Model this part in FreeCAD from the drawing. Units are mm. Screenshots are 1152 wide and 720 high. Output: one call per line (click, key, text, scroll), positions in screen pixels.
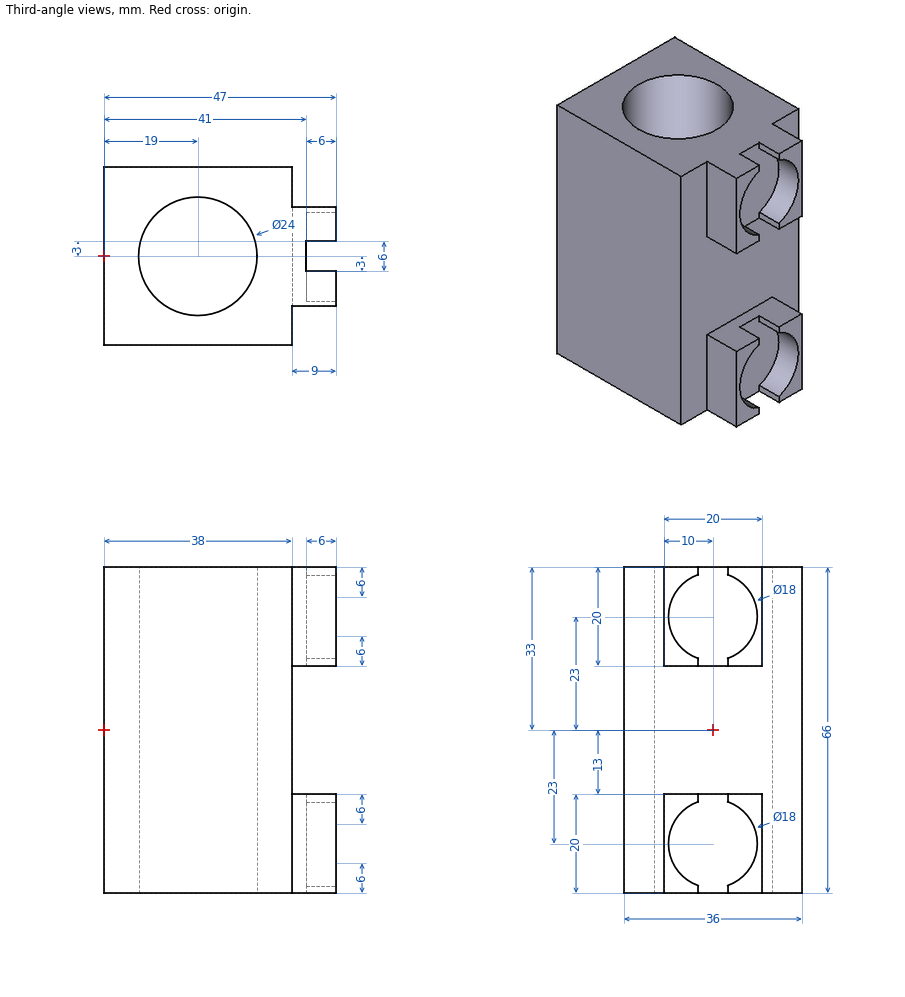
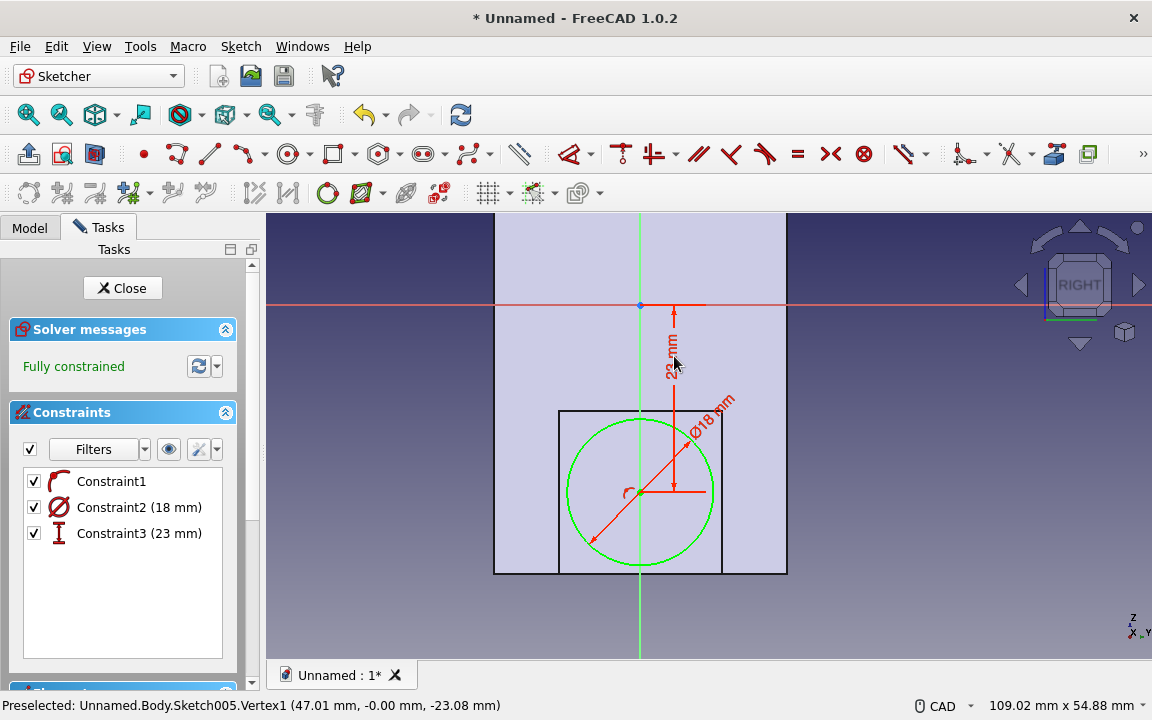
click(123, 288)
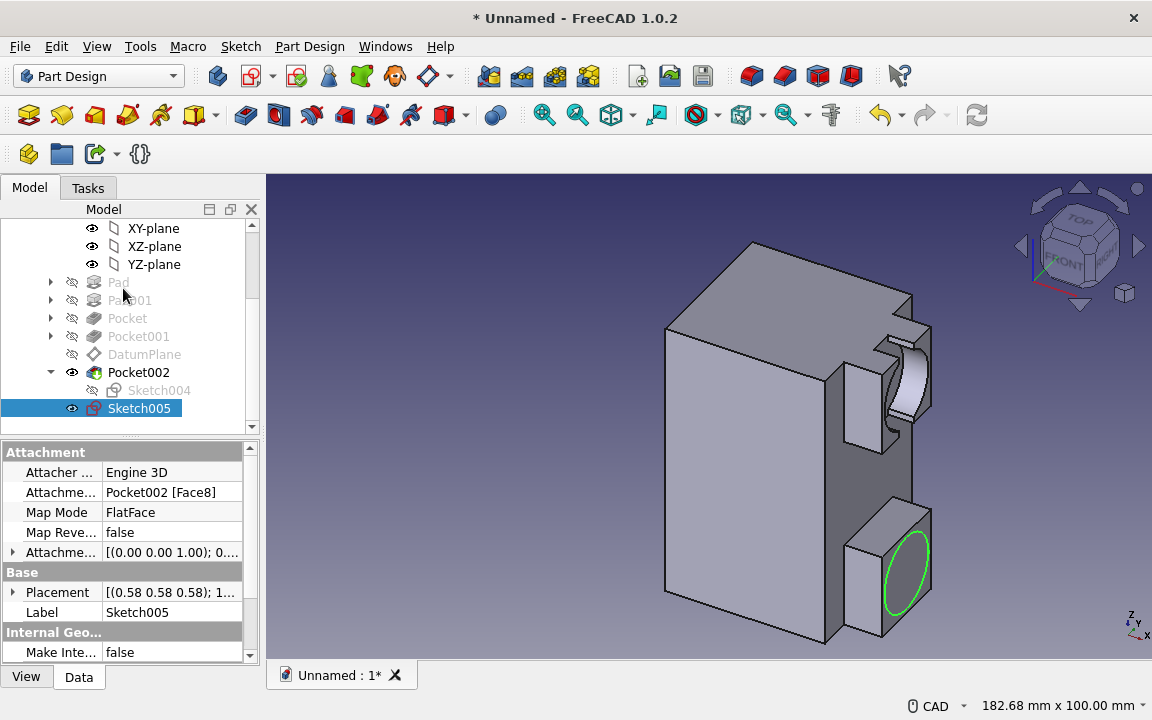
click(246, 116)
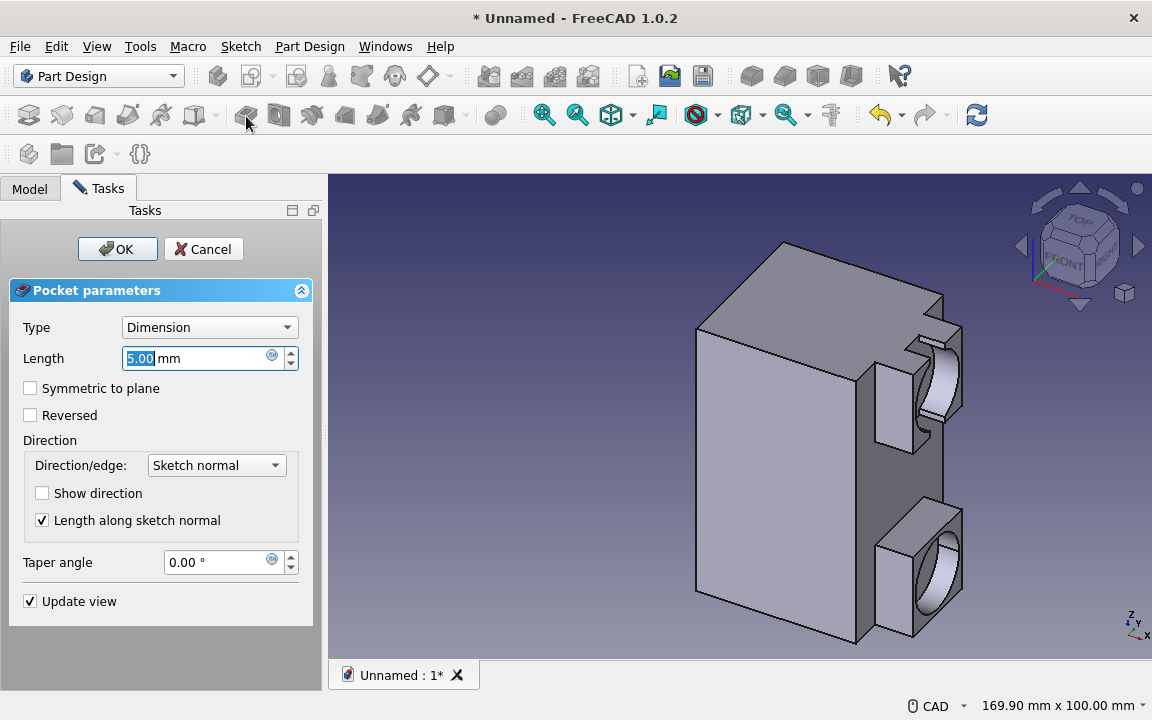
text(6)
key(Tab)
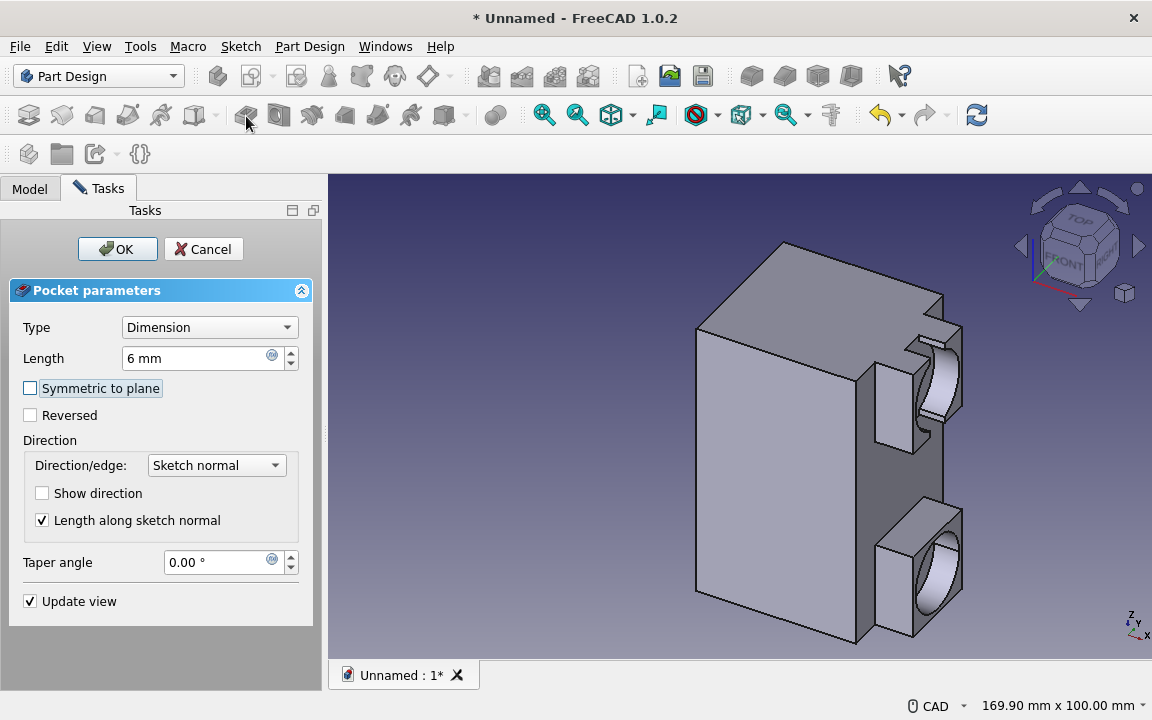
click(118, 249)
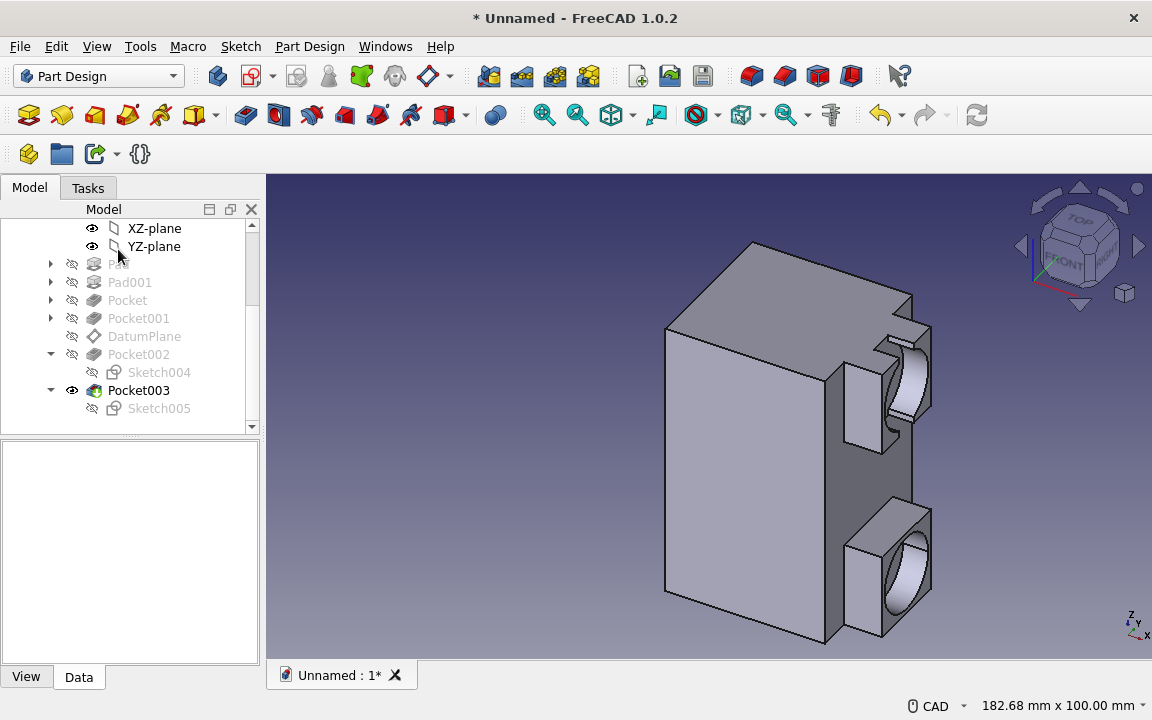
key(5)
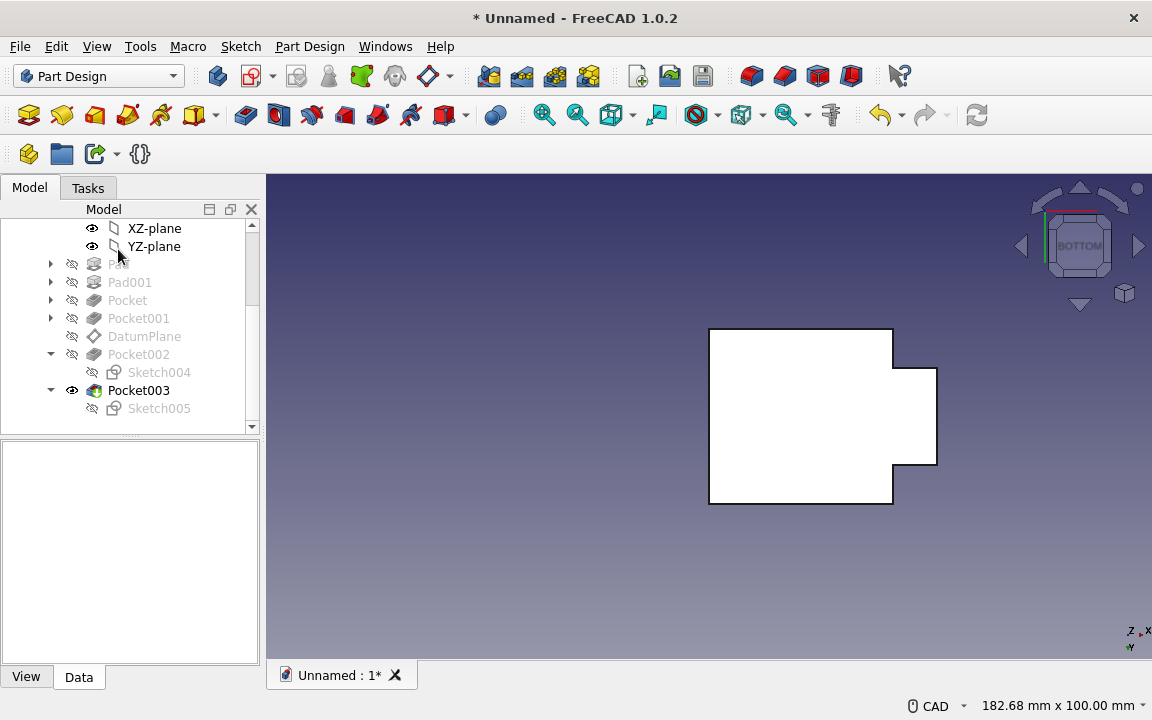
click(545, 116)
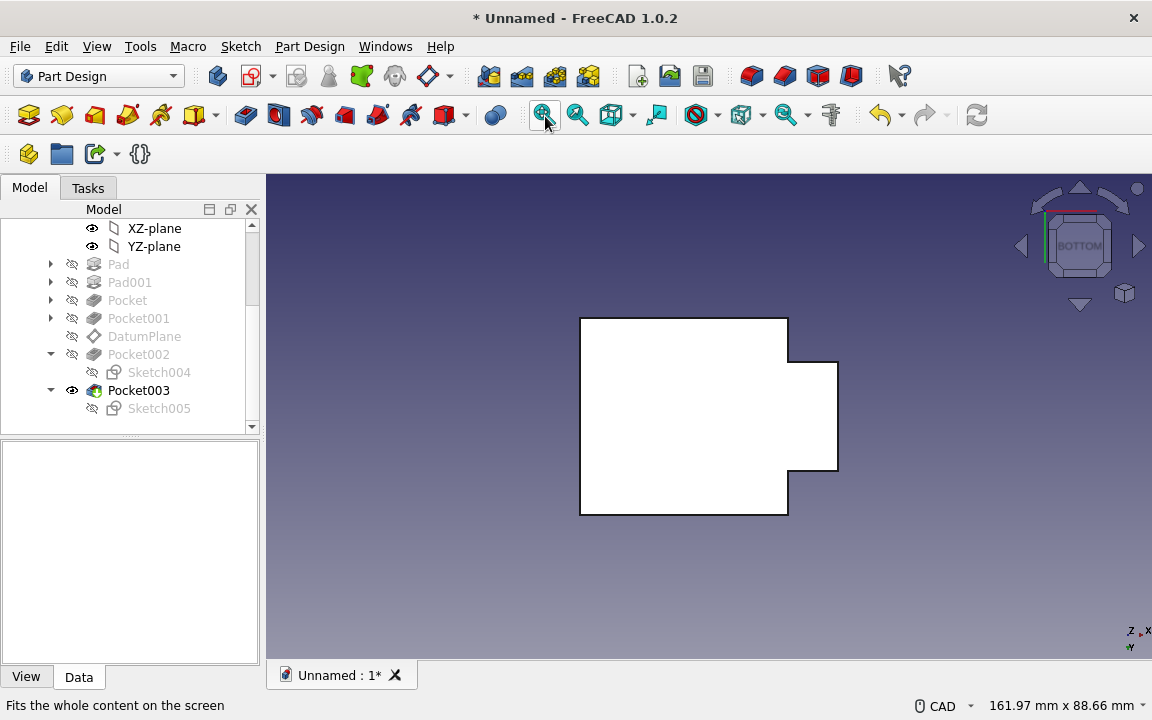
click(709, 415)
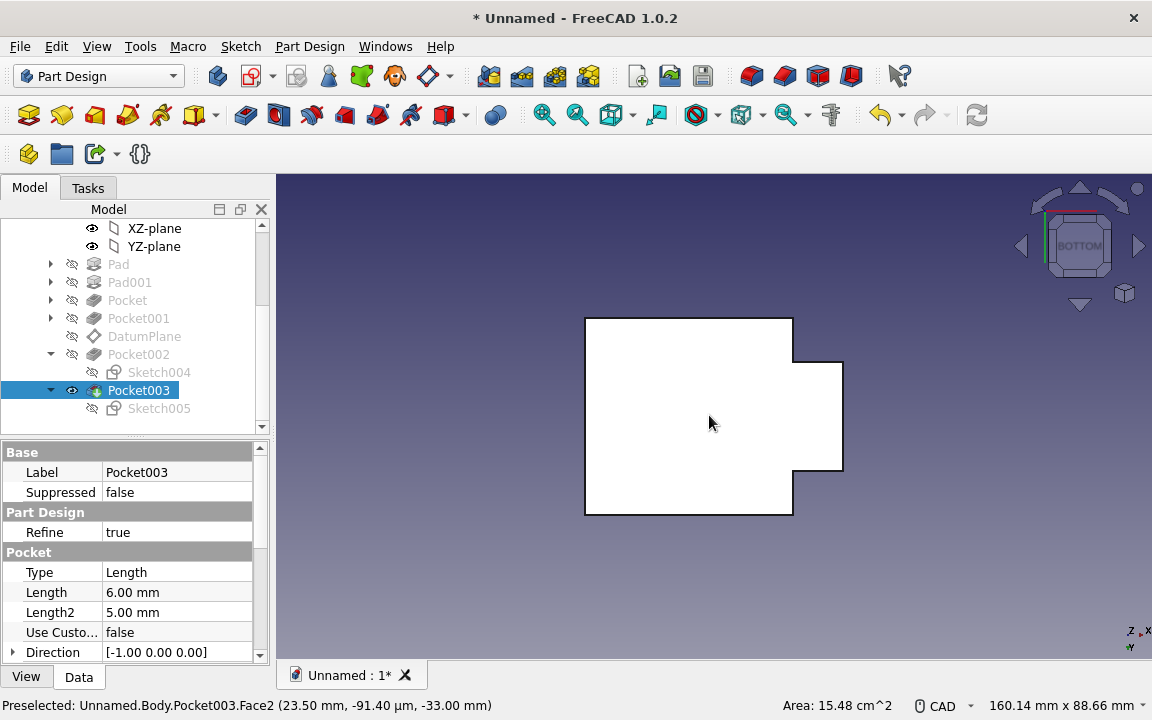
click(250, 76)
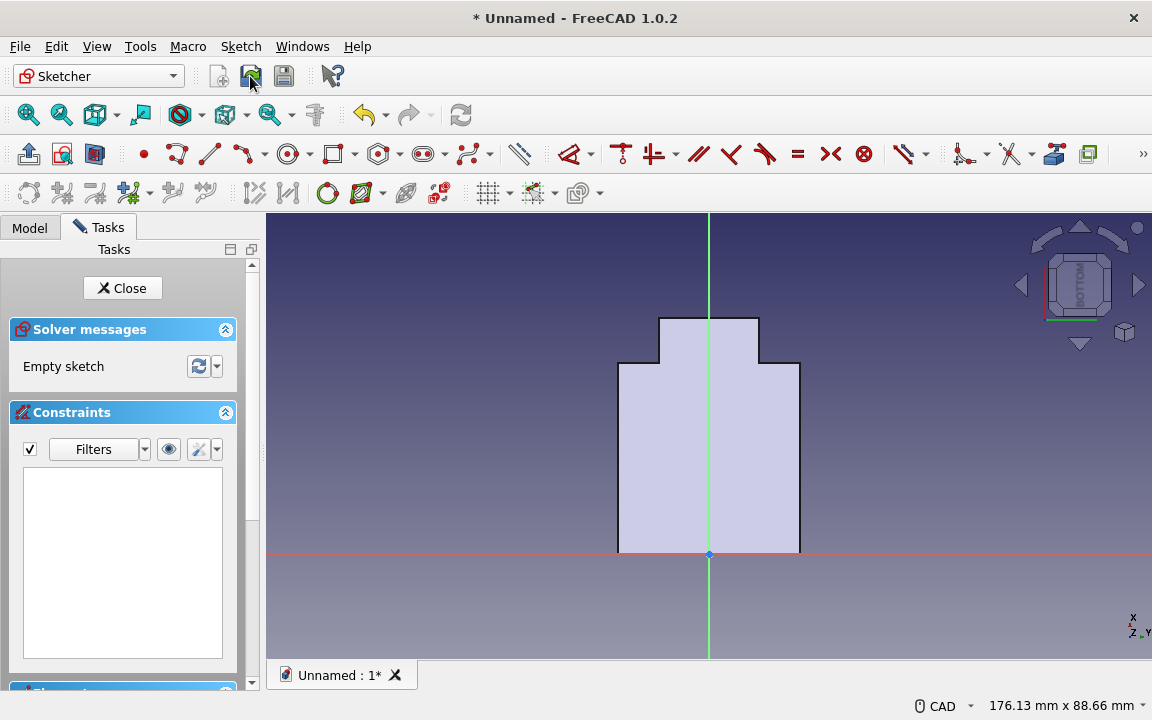
scroll(718, 320, up, 11)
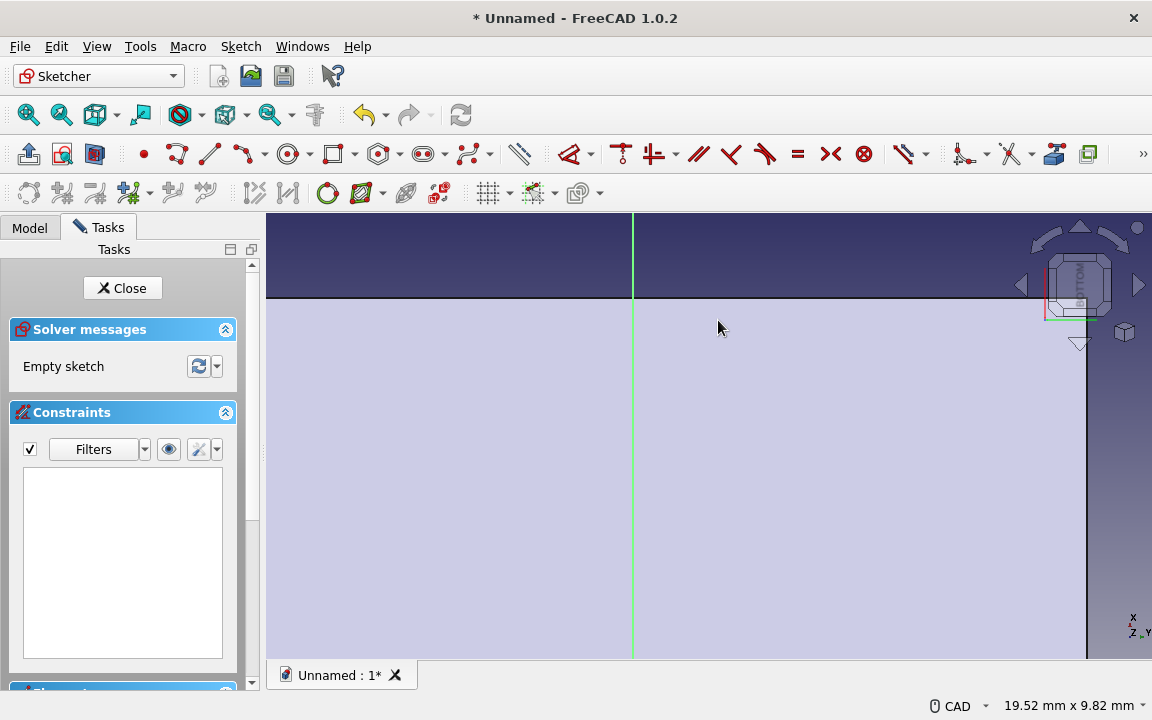
click(332, 154)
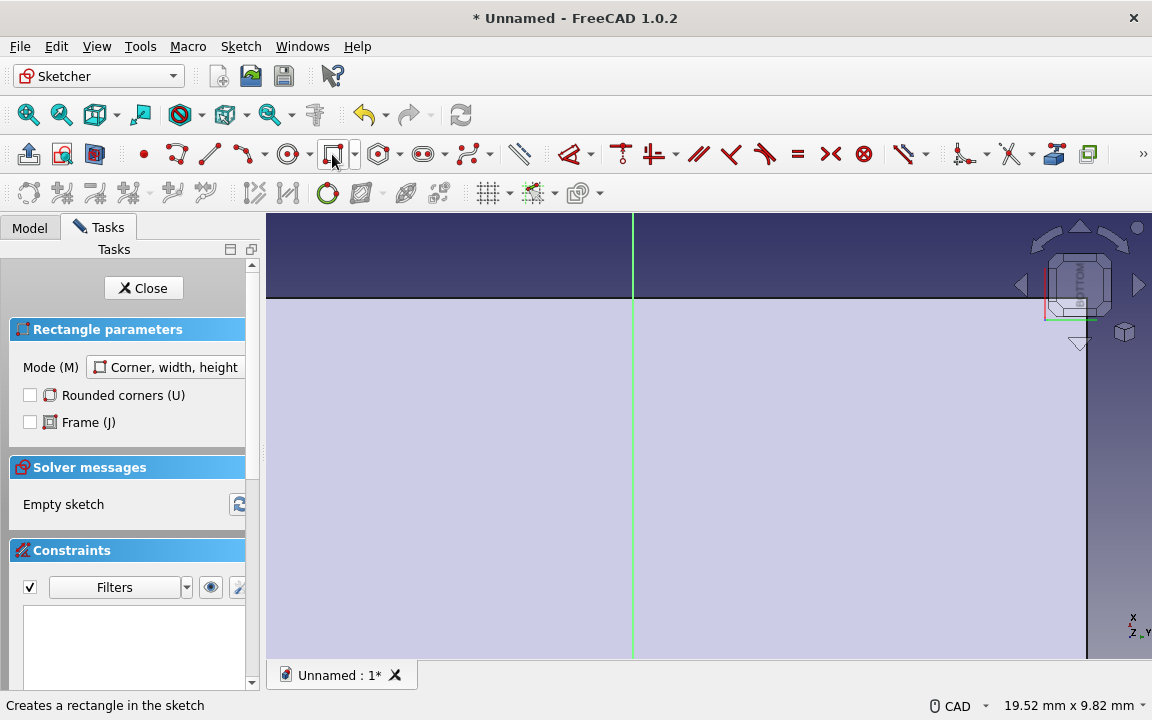
click(496, 298)
click(769, 570)
key(Escape)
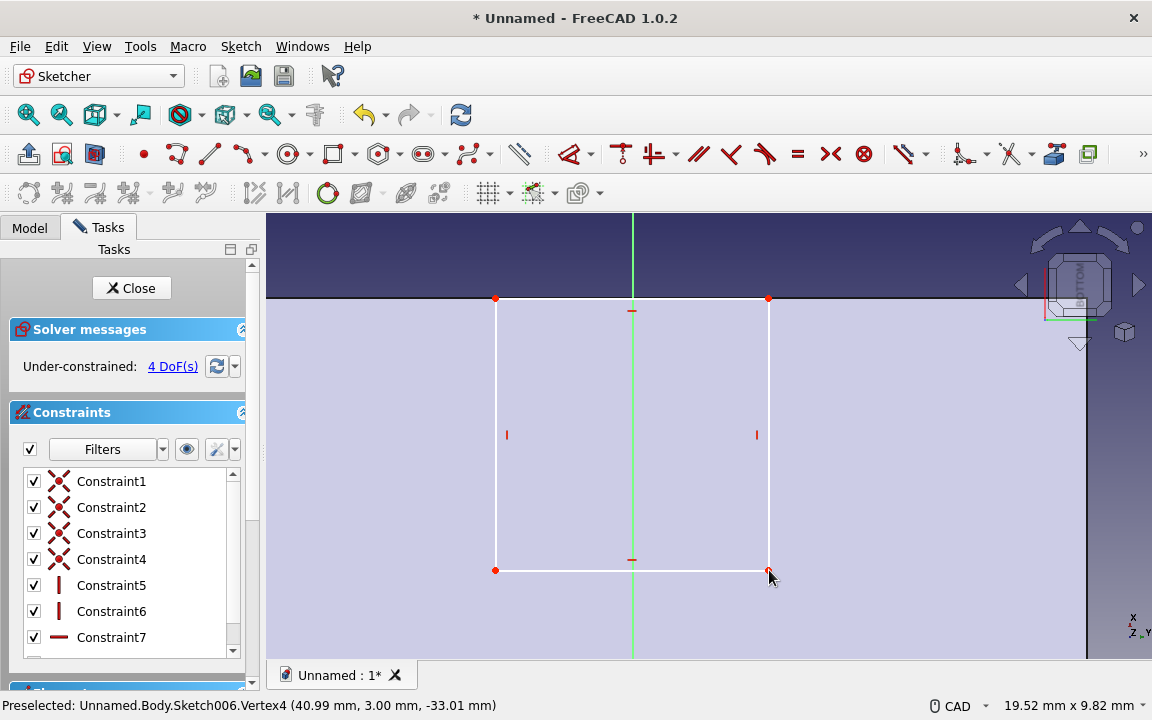
key(d)